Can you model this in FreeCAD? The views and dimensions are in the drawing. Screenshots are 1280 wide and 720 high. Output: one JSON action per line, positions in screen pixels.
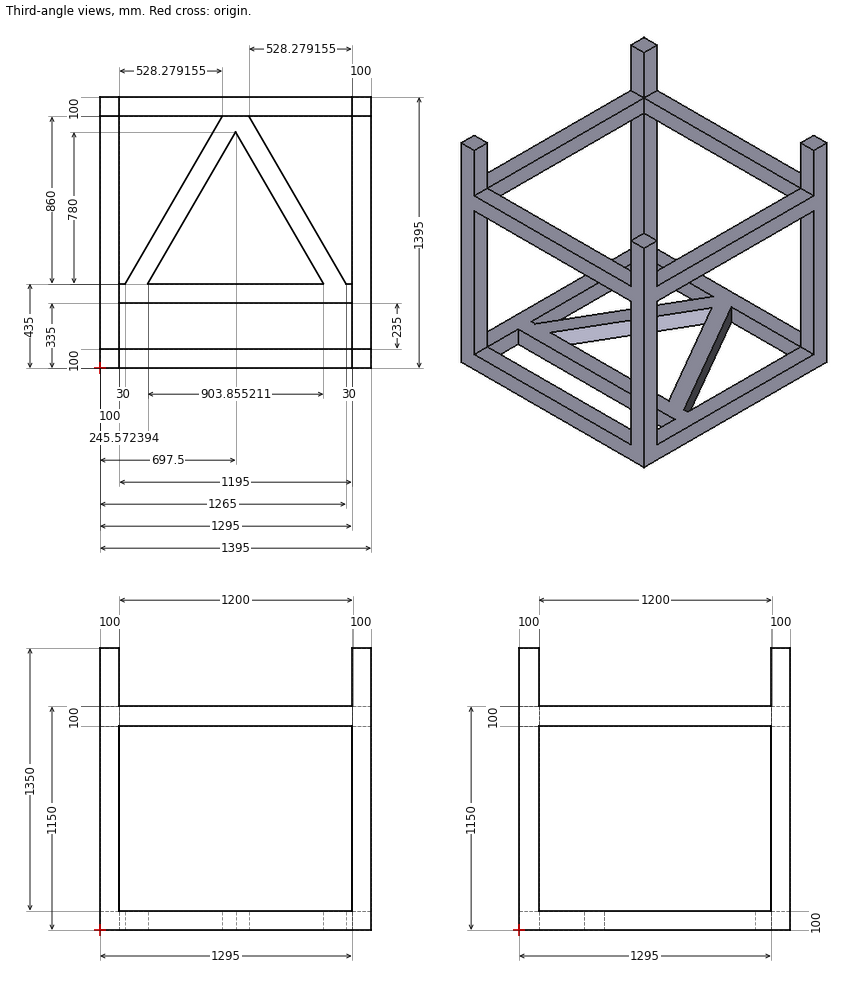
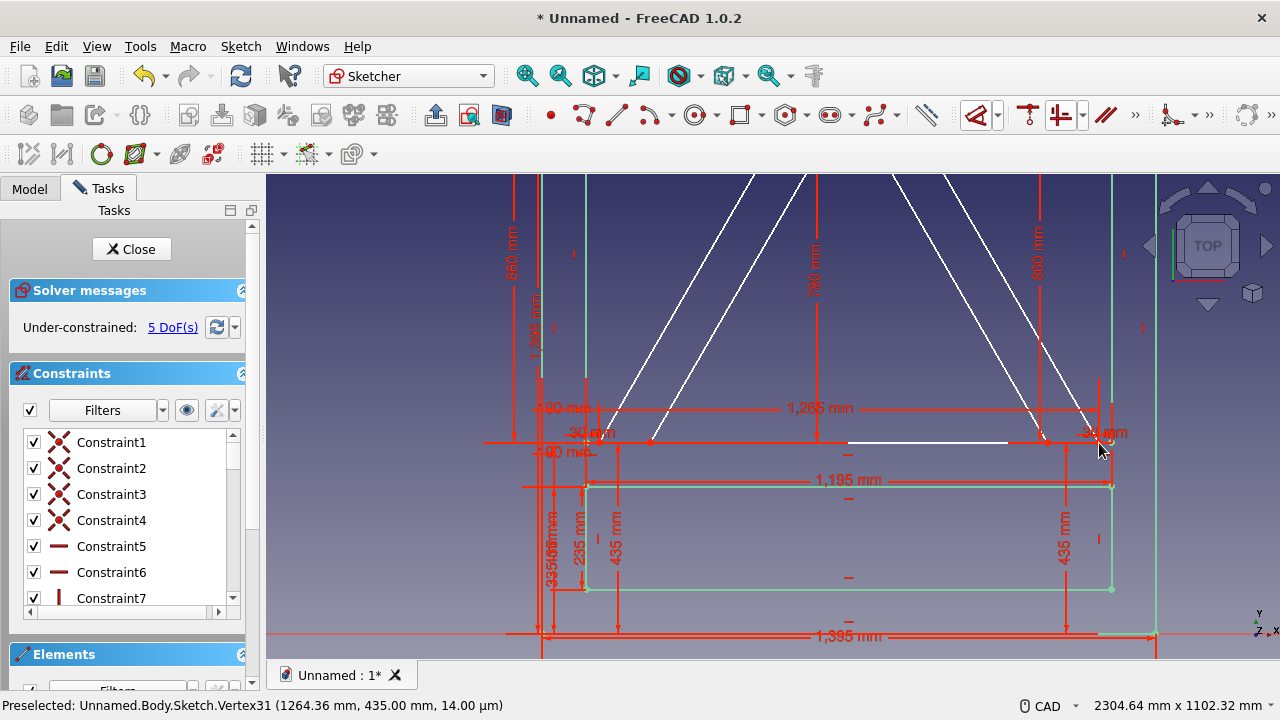
{"action": "scroll", "coordinate": [587, 489], "scroll_direction": "down", "scroll_amount": 4}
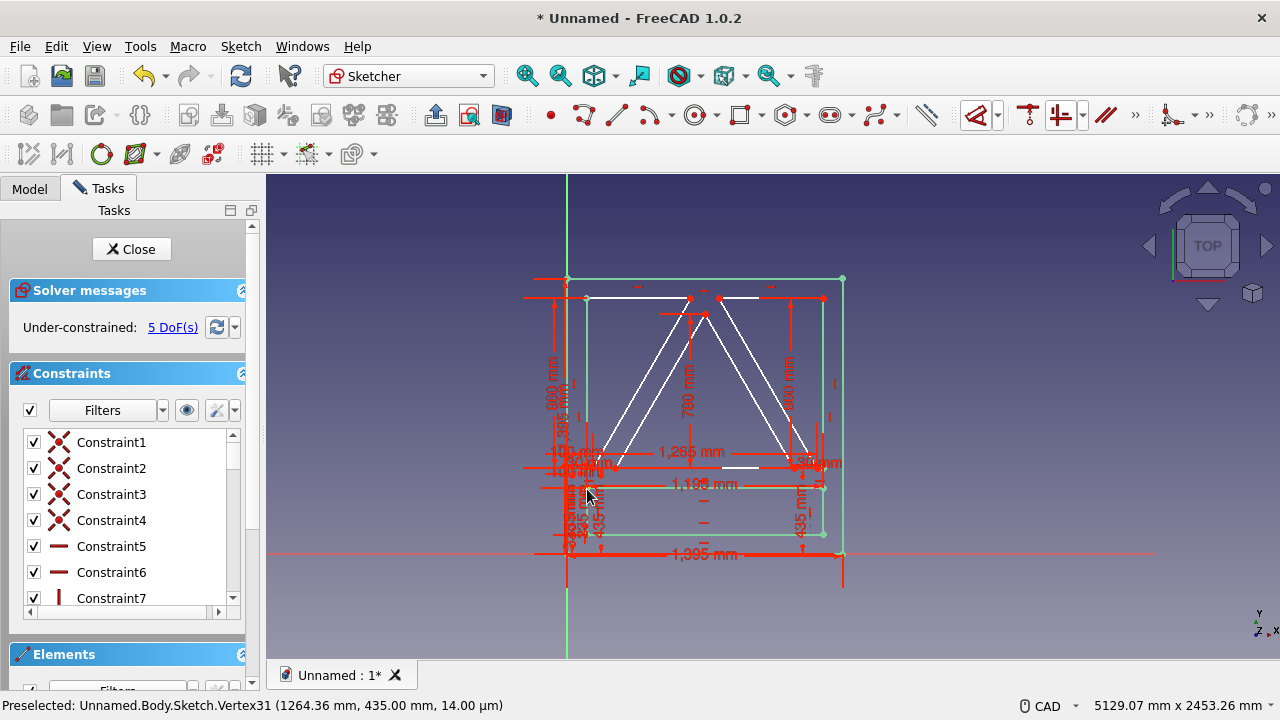
{"action": "left_click", "coordinate": [705, 314]}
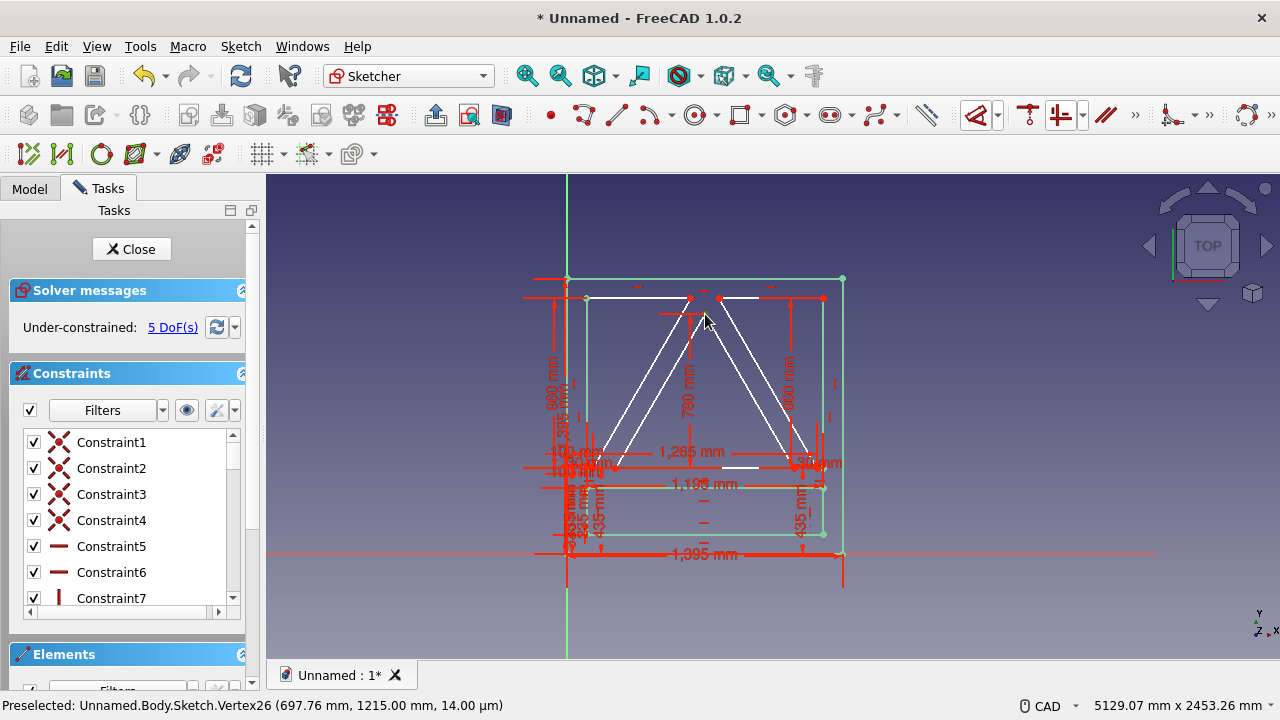
{"action": "key", "text": "l"}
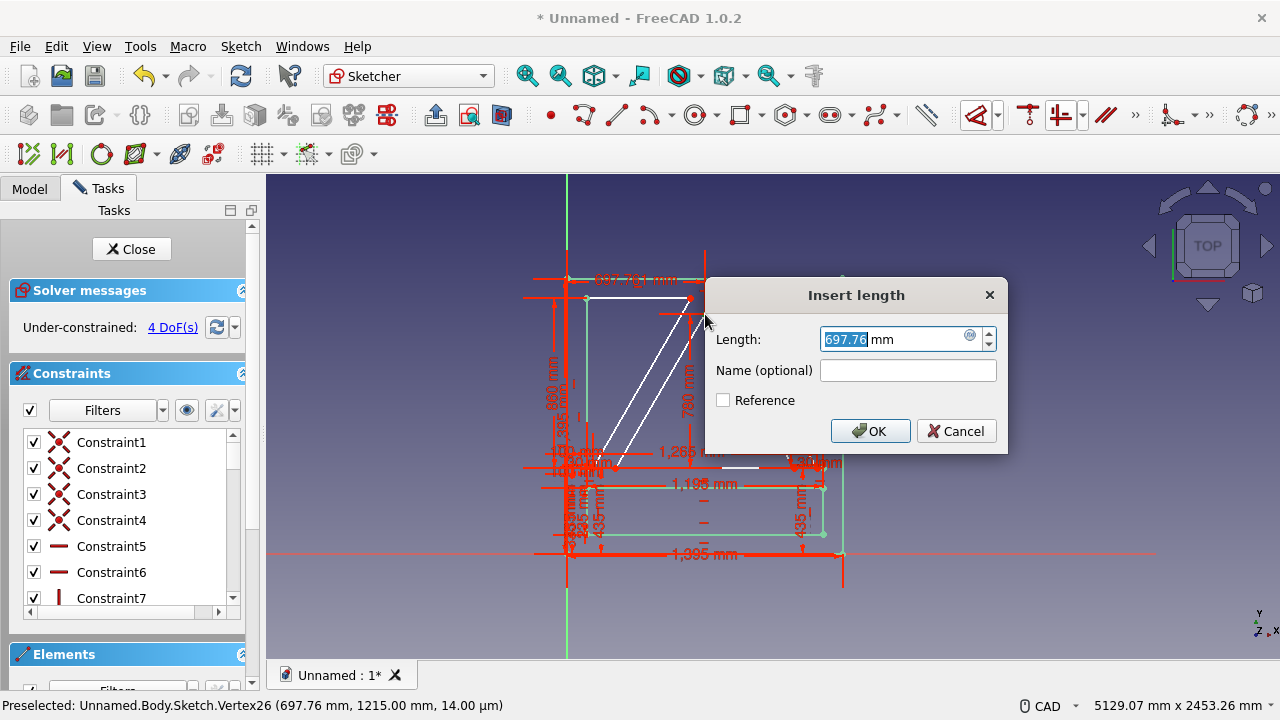
{"action": "type", "text": "697.5"}
{"action": "key", "text": "Return"}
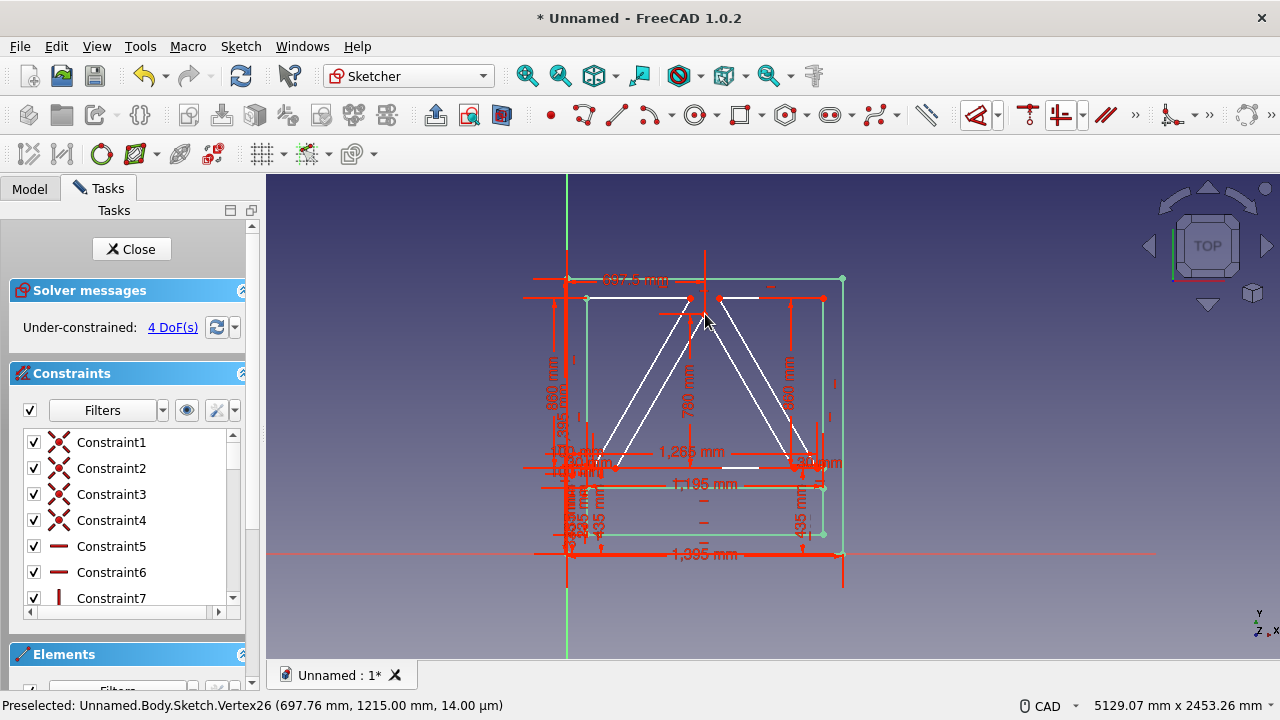
{"action": "left_click", "coordinate": [618, 298]}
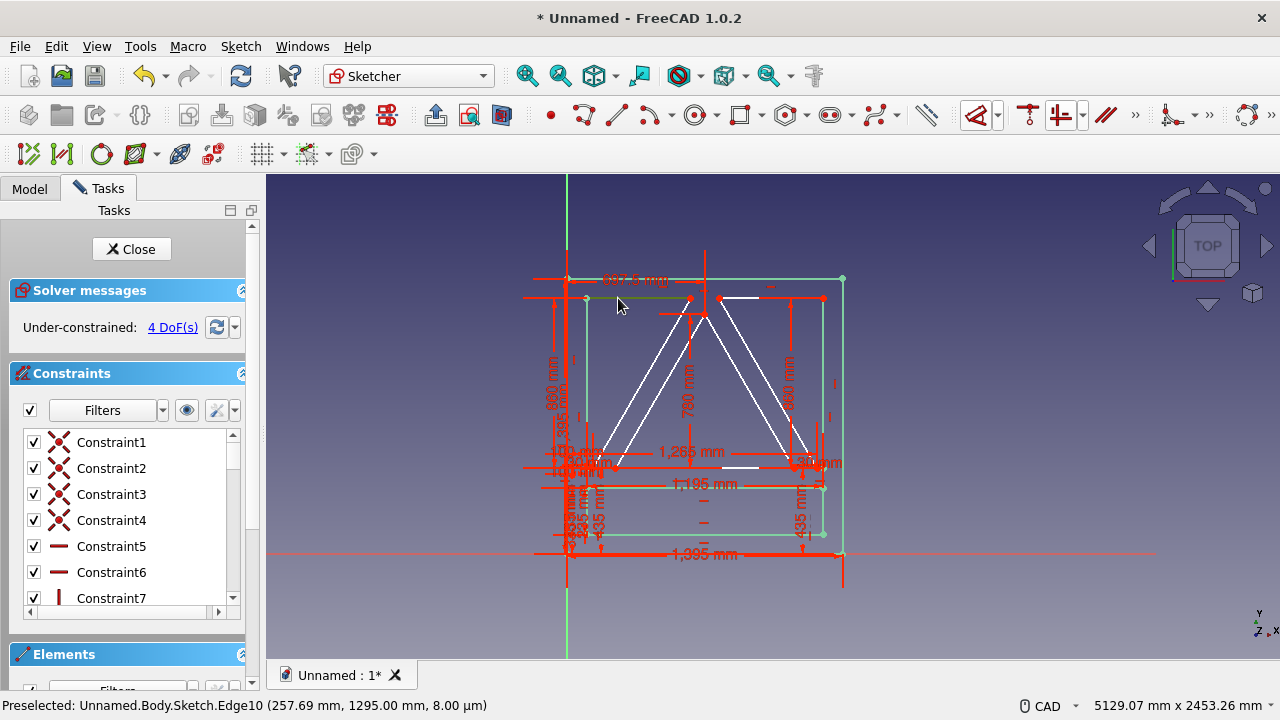
{"action": "key", "text": "l"}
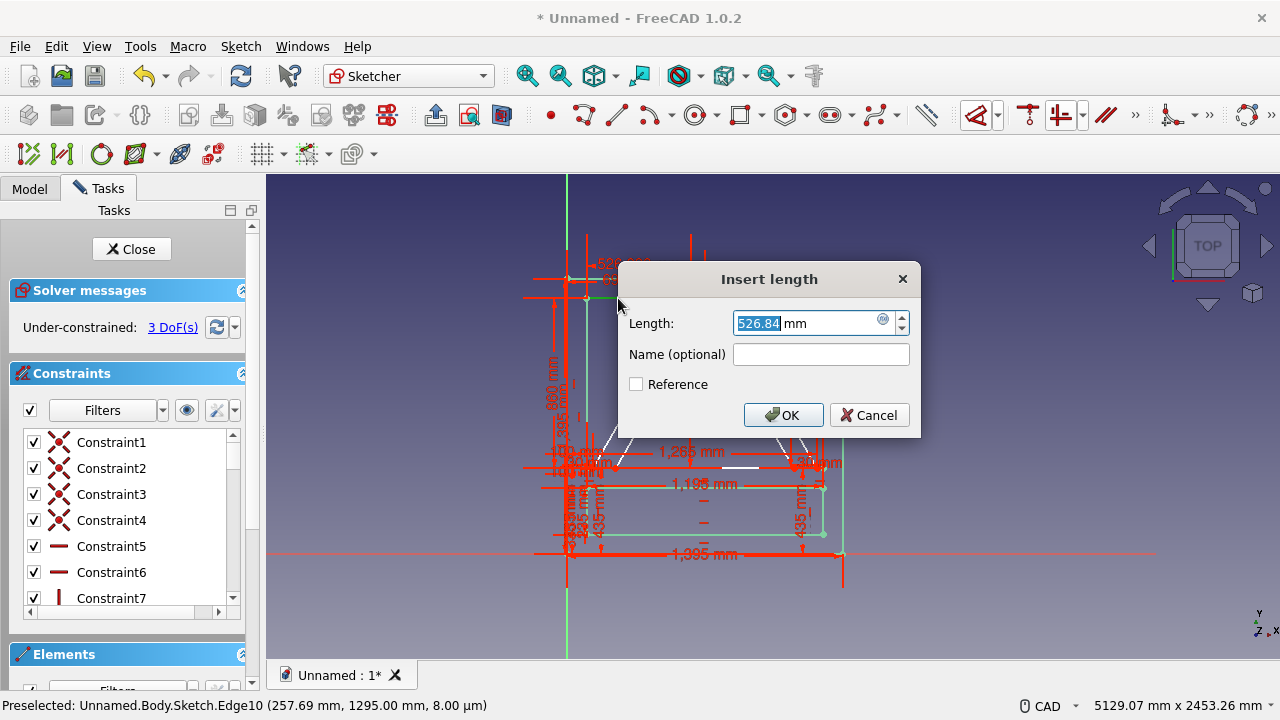
{"action": "type", "text": "528.279155"}
{"action": "key", "text": "Return"}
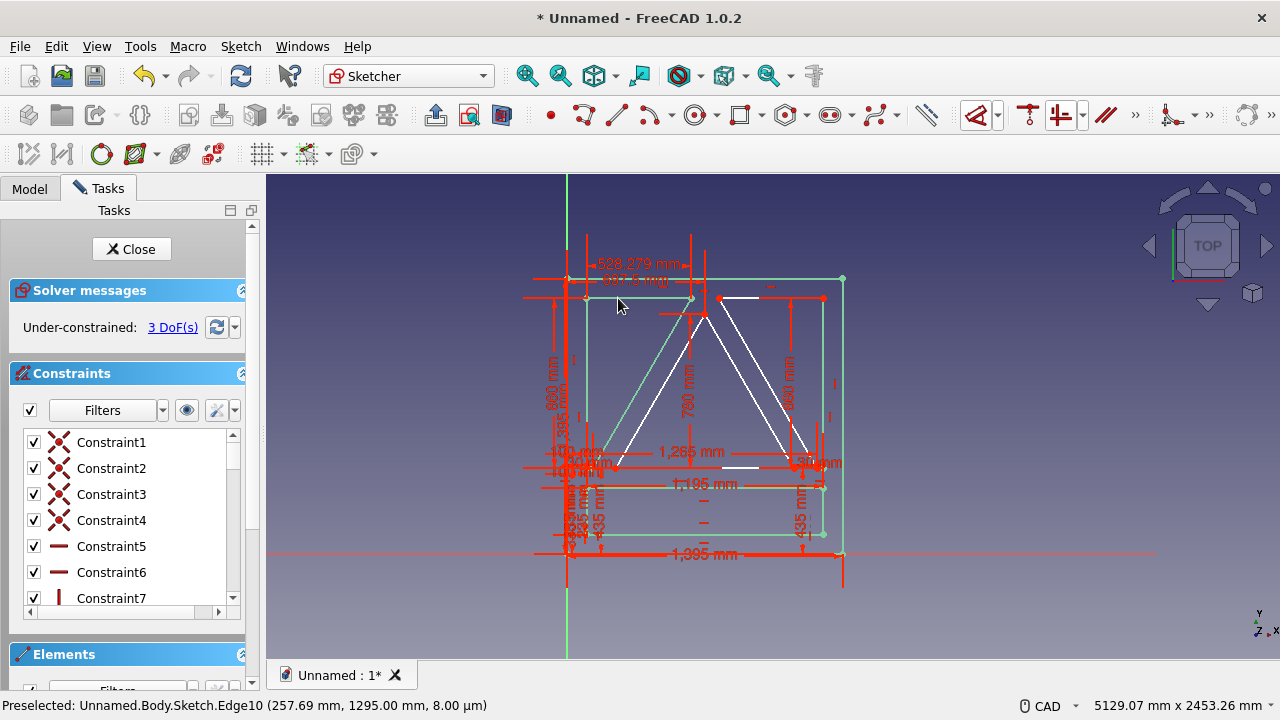
{"action": "left_click", "coordinate": [741, 468]}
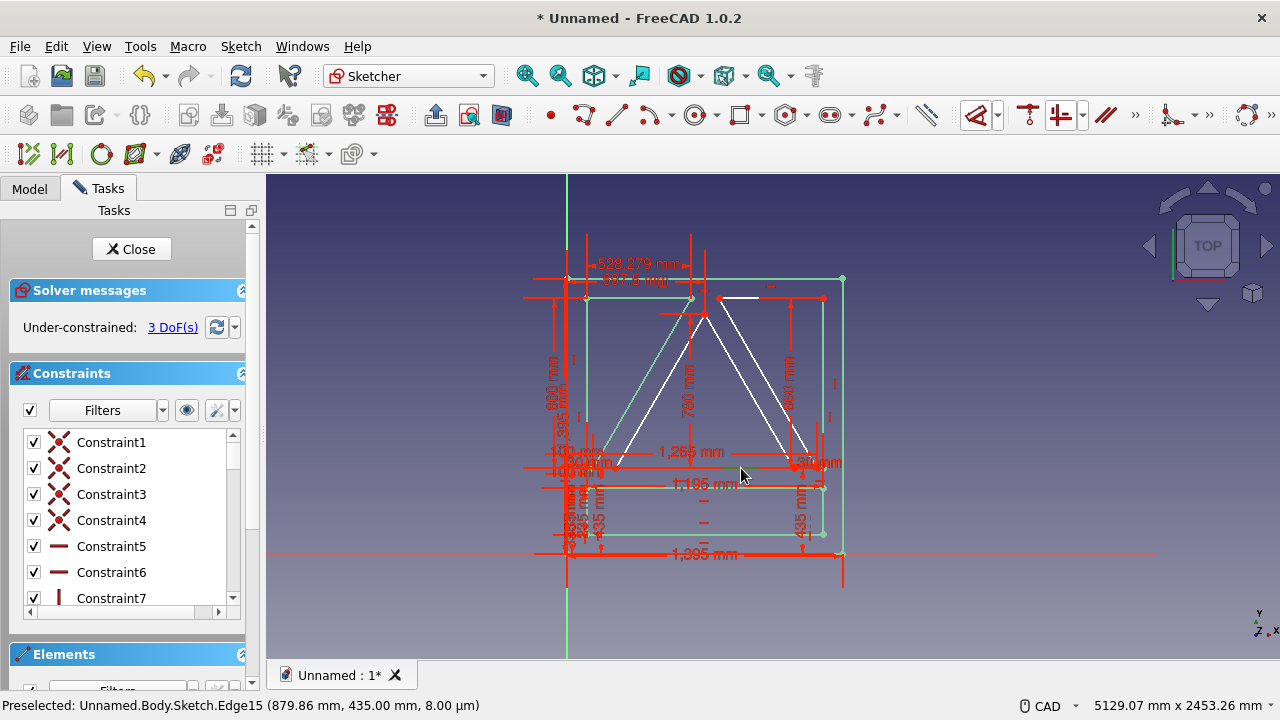
{"action": "key", "text": "l"}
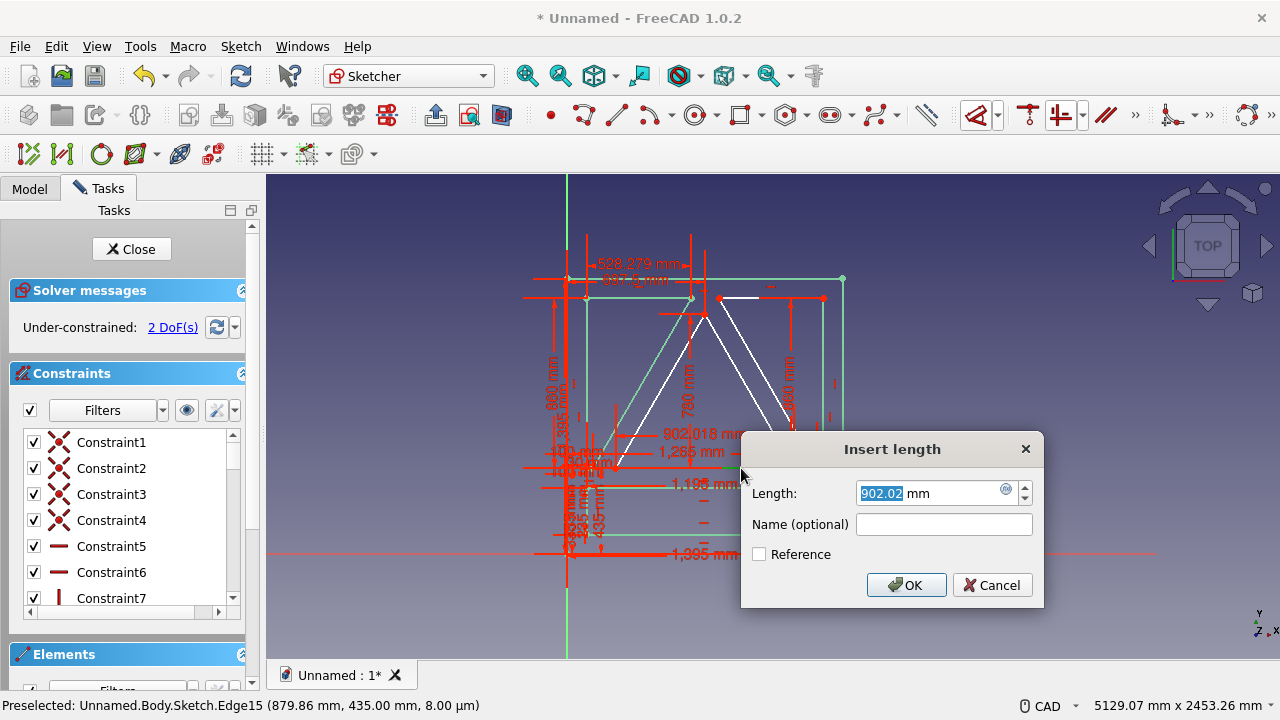
{"action": "type", "text": "903.855211"}
{"action": "key", "text": "Return"}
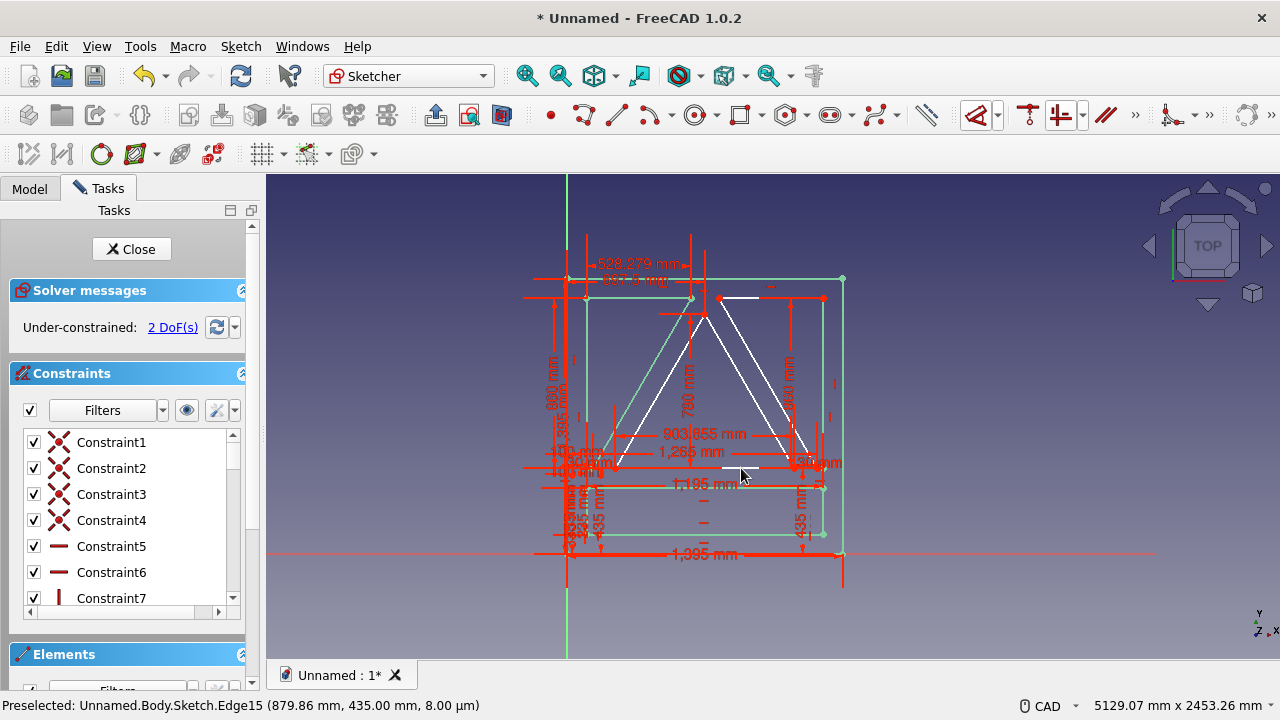
{"action": "left_click", "coordinate": [750, 298]}